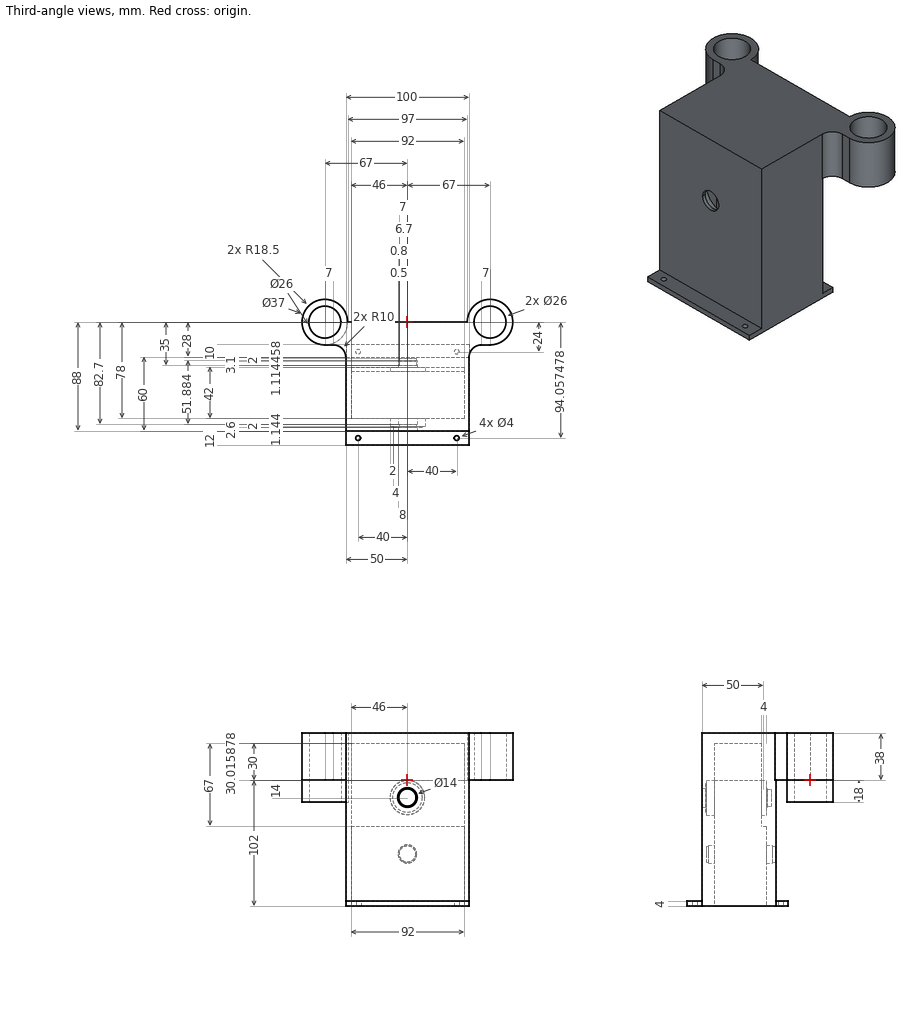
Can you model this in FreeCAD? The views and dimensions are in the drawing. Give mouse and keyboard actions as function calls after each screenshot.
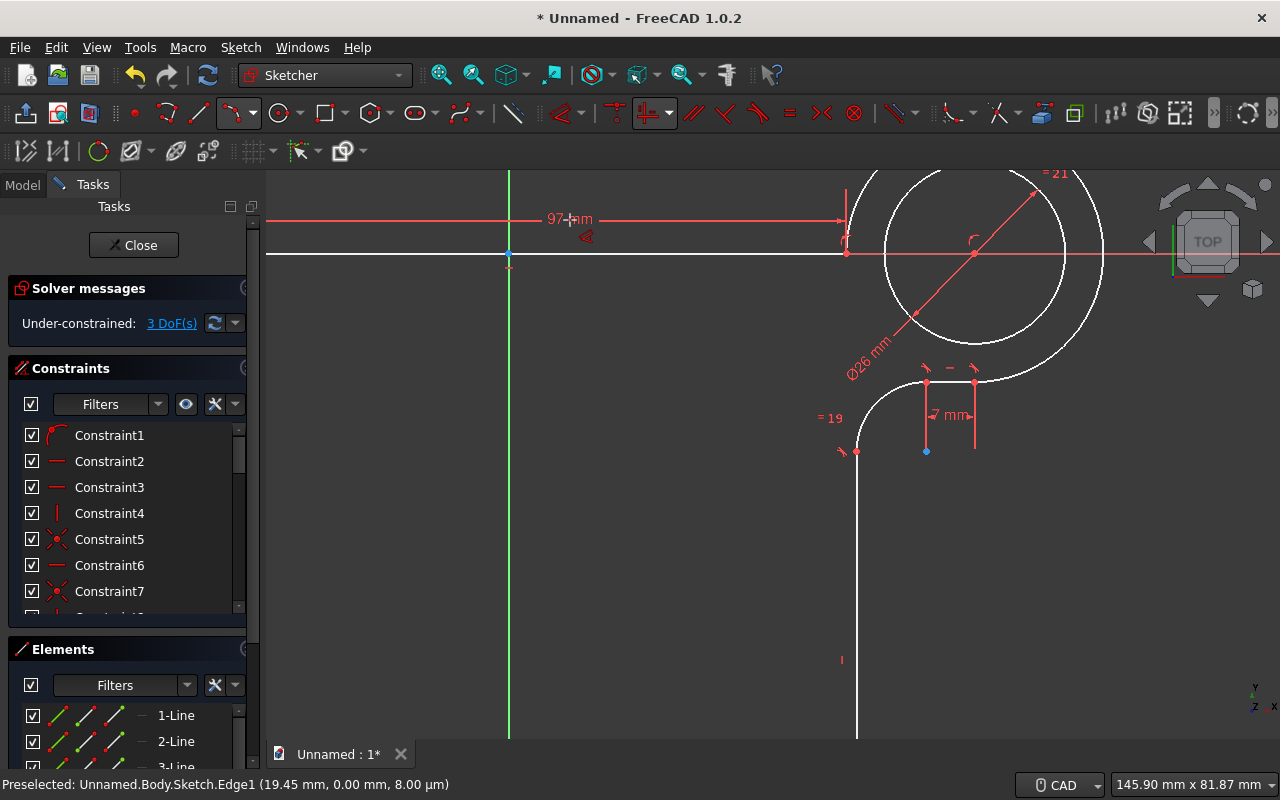
click(975, 254)
click(742, 220)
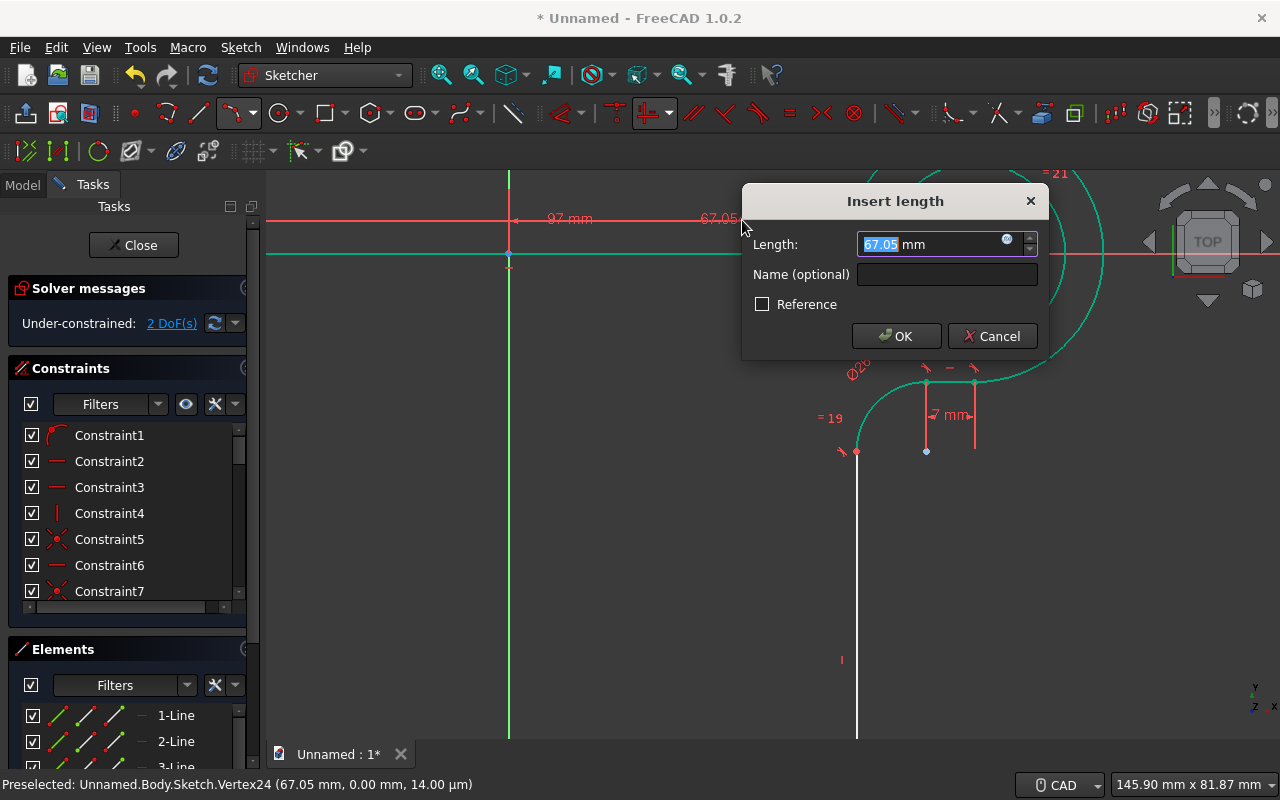
text(67)
key(Return)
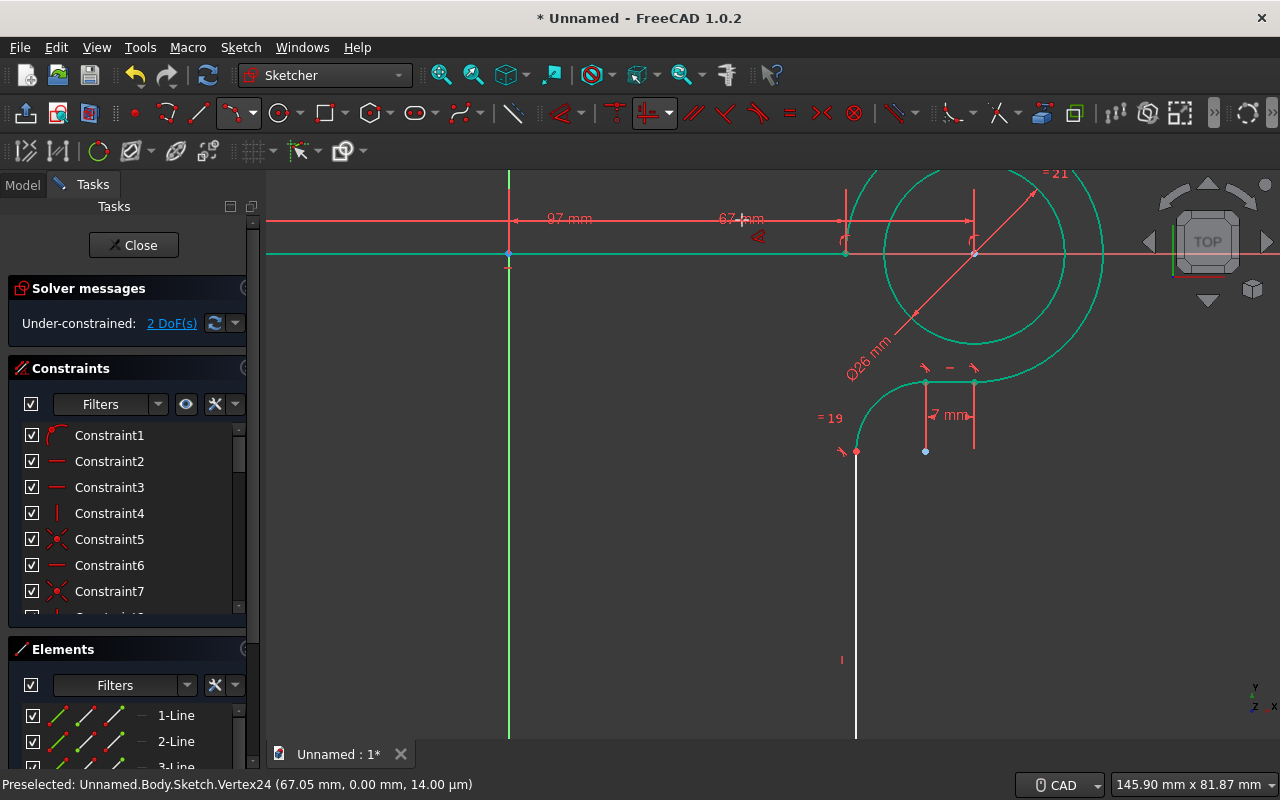
scroll(943, 382, down, 3)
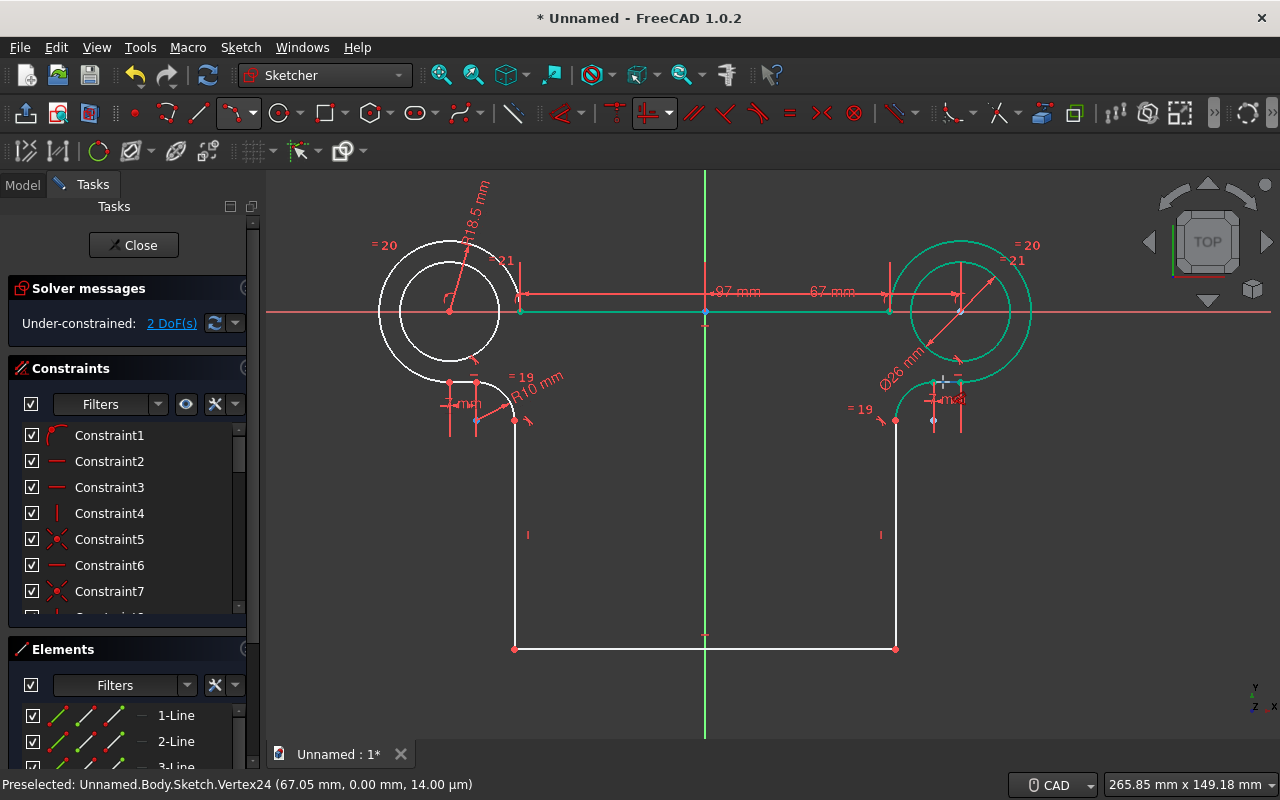
click(450, 312)
click(577, 278)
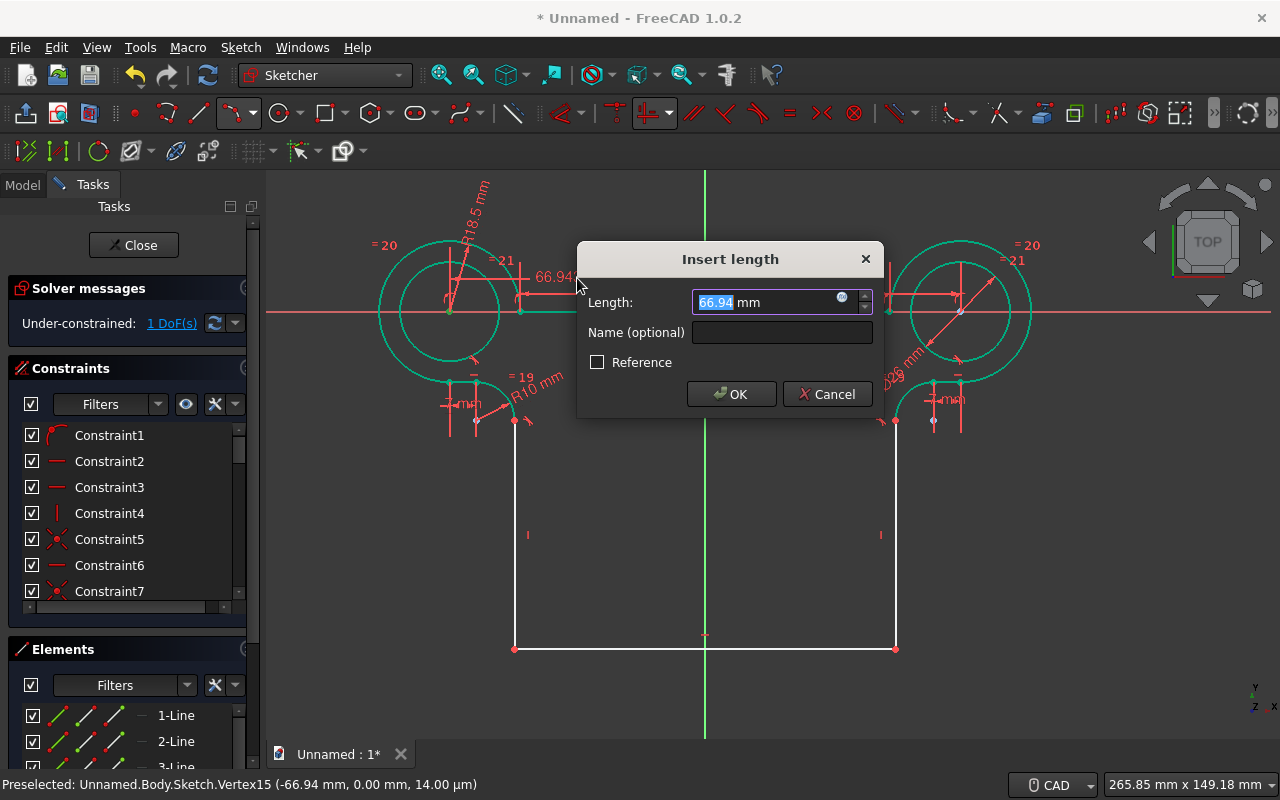
text(67)
key(Return)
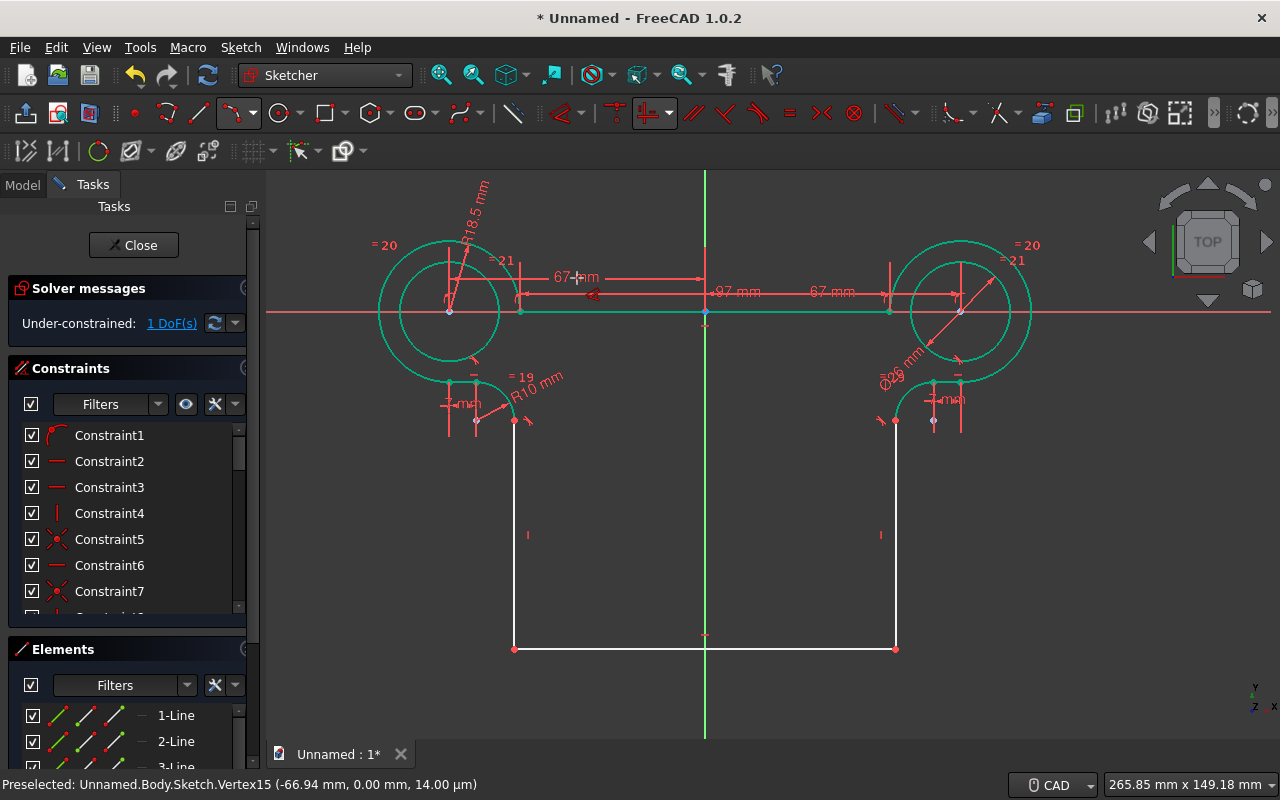
click(514, 649)
click(480, 480)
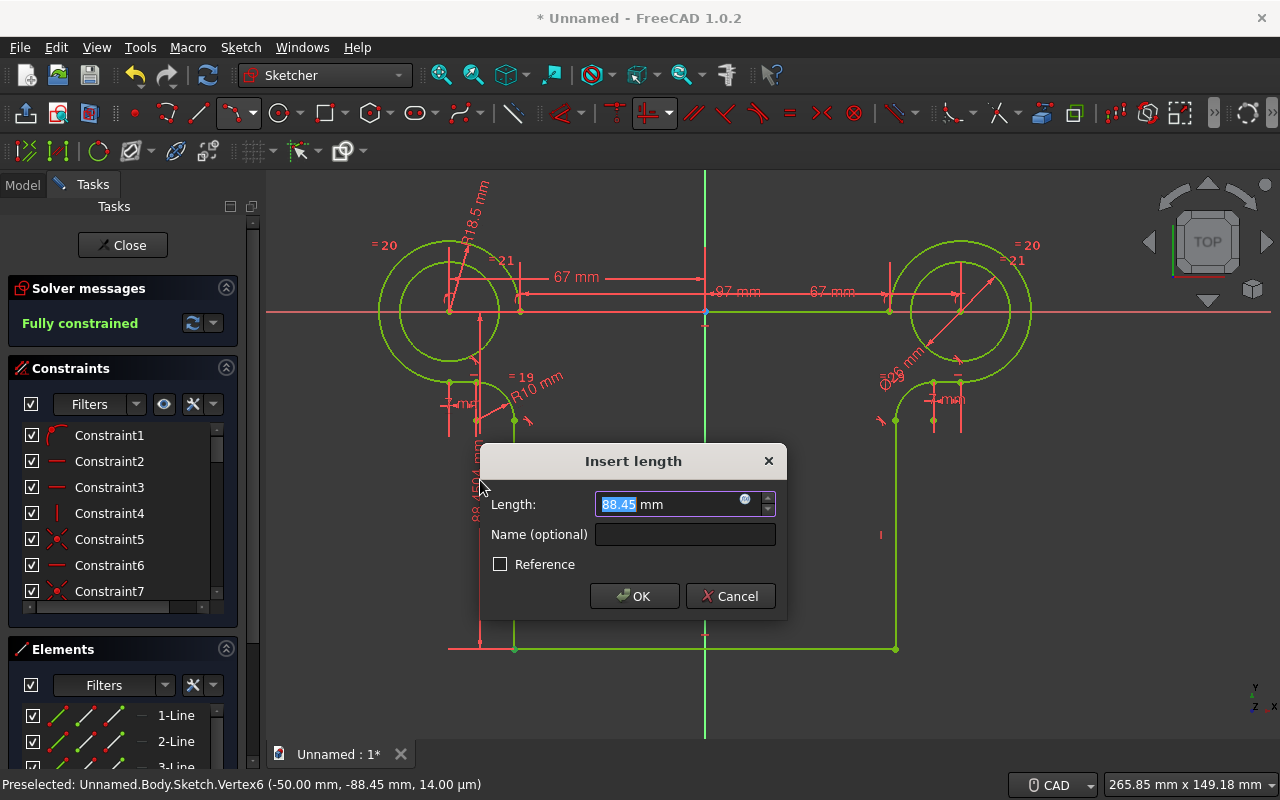
text(88)
key(Return)
key(Escape)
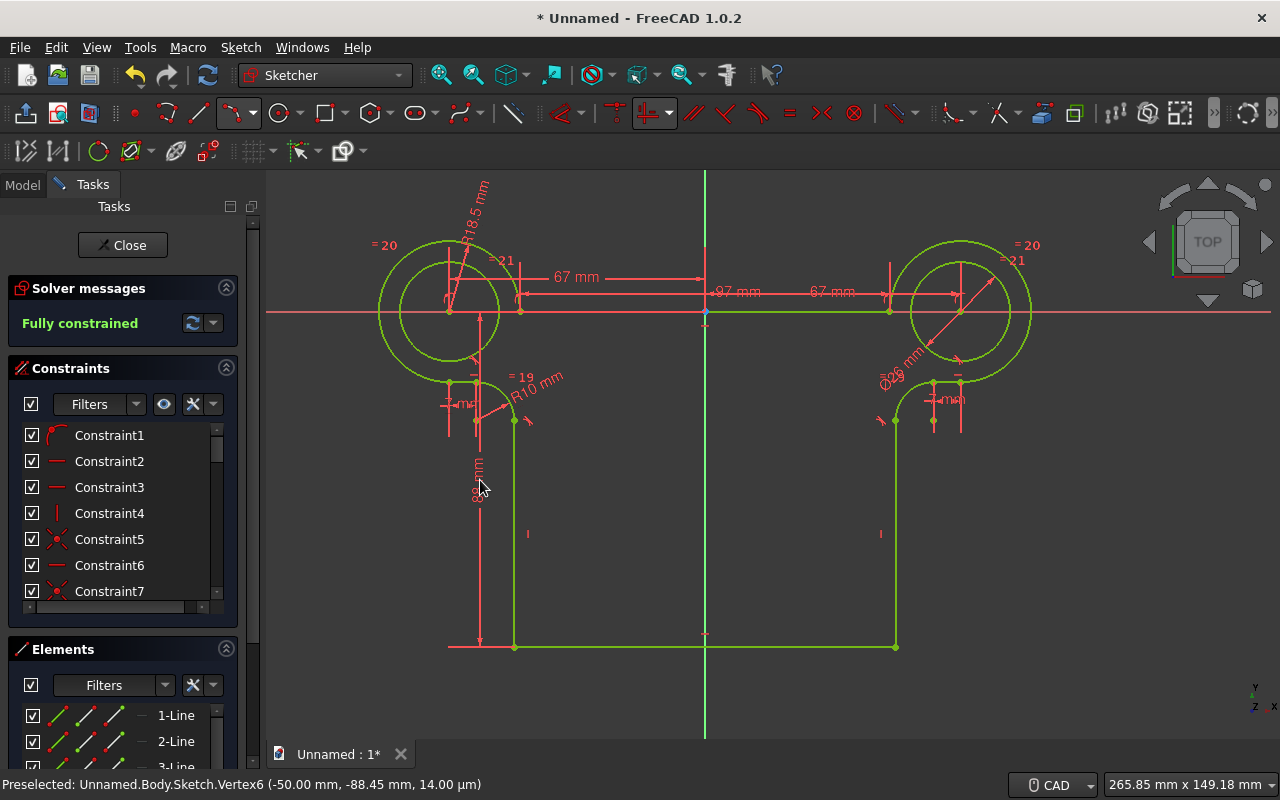
click(123, 245)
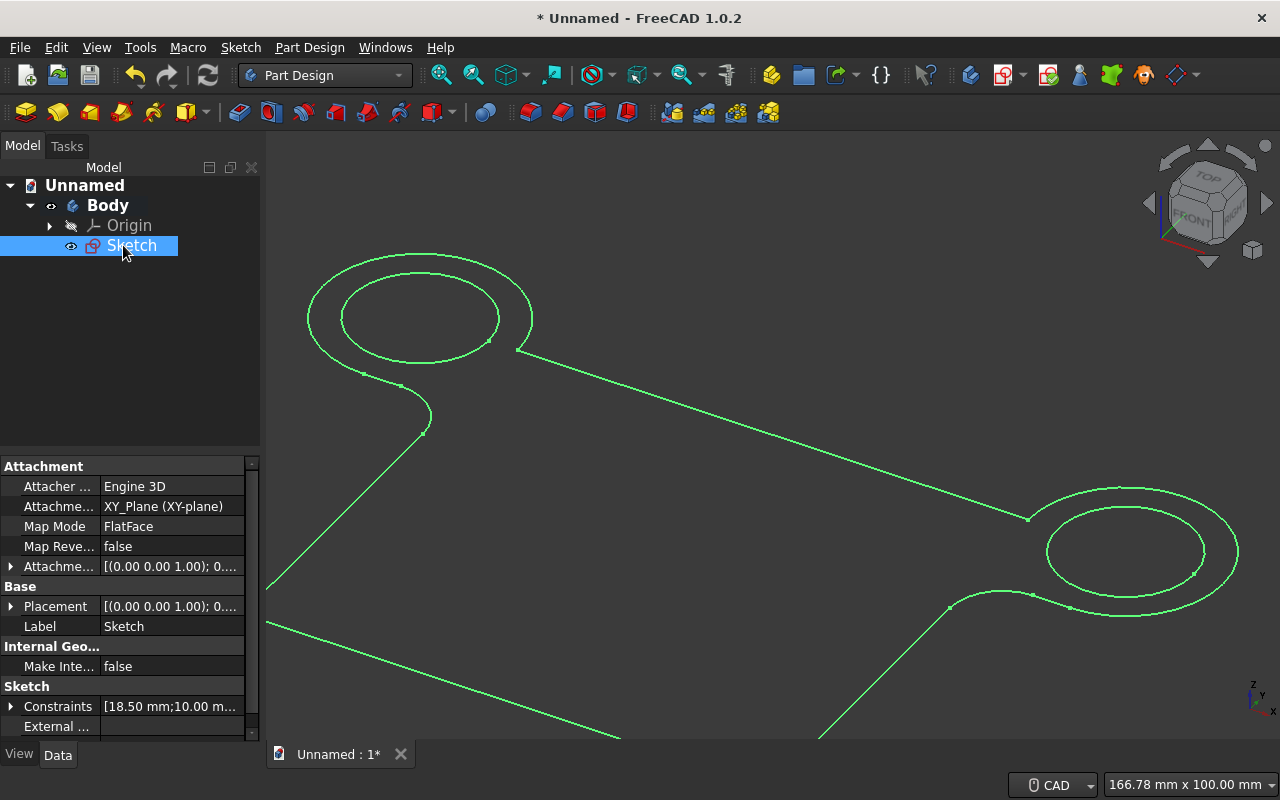
click(26, 112)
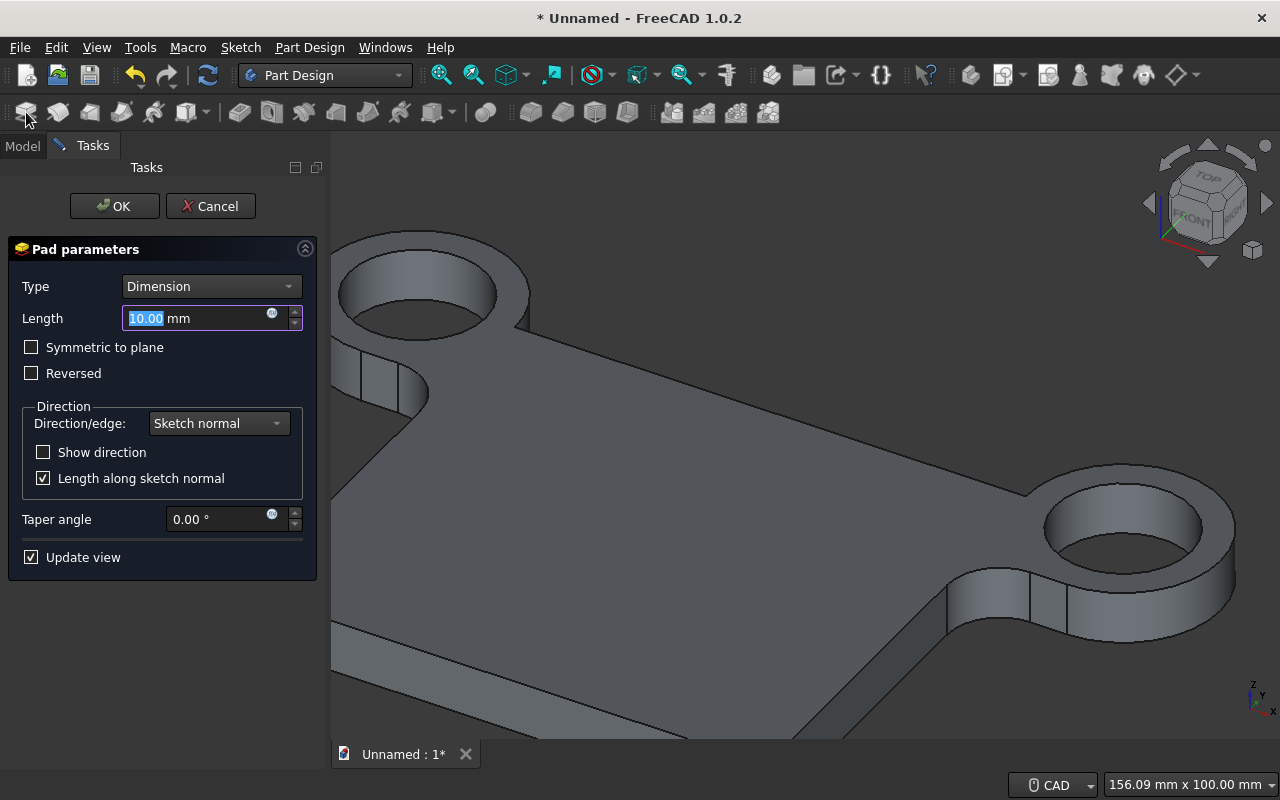
text(38)
key(Tab)